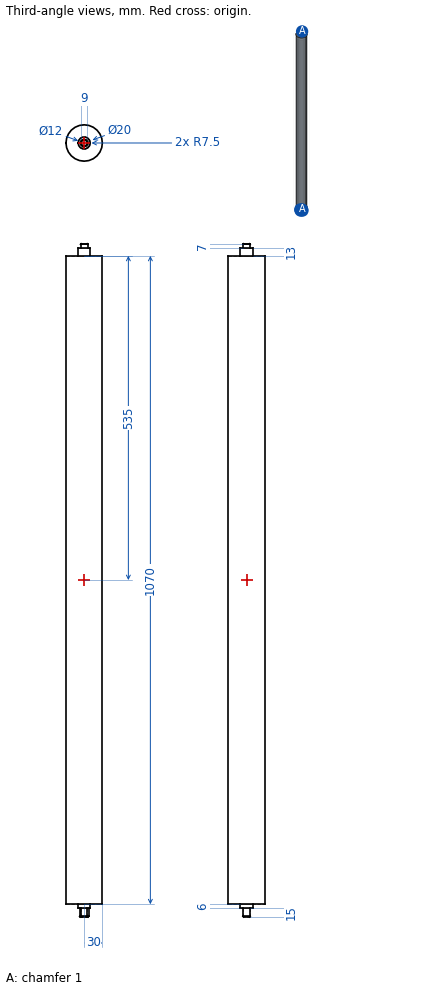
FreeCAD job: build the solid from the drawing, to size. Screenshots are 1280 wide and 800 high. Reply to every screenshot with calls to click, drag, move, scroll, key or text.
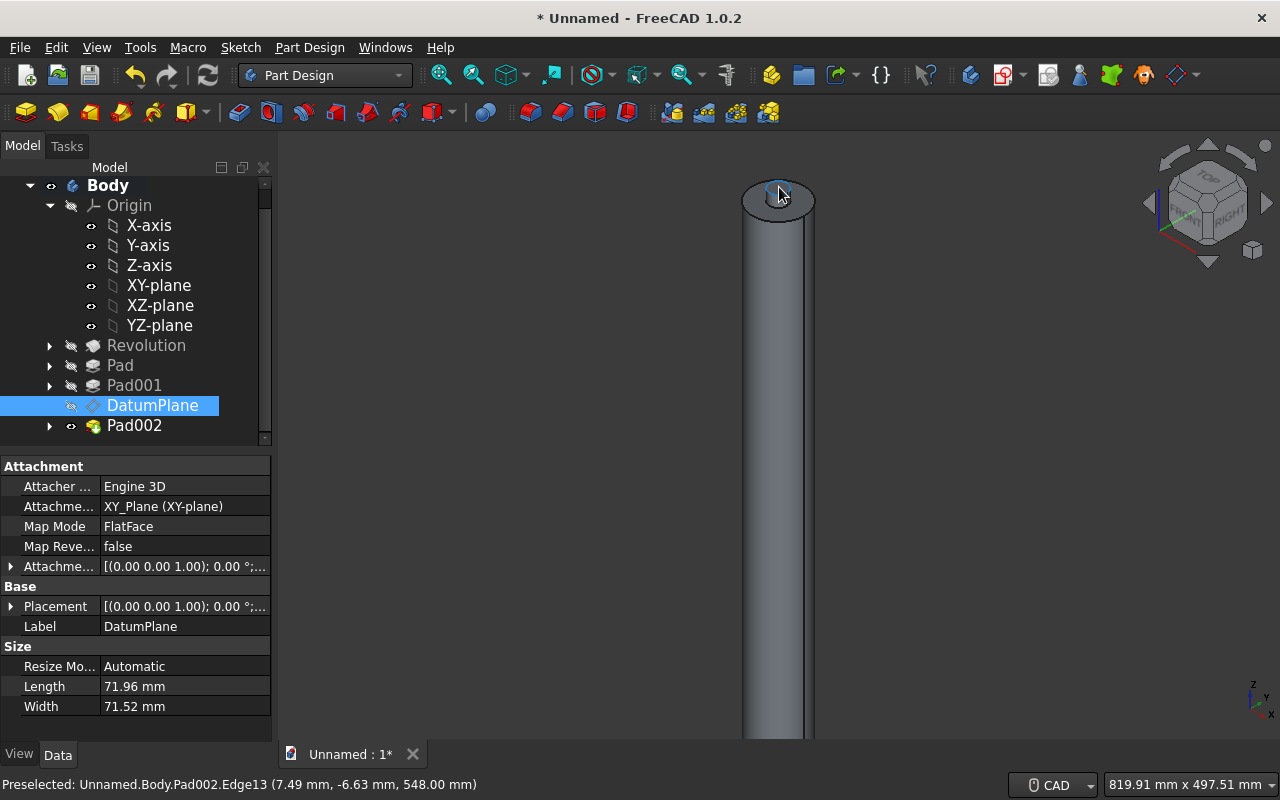
key(v)
key(f)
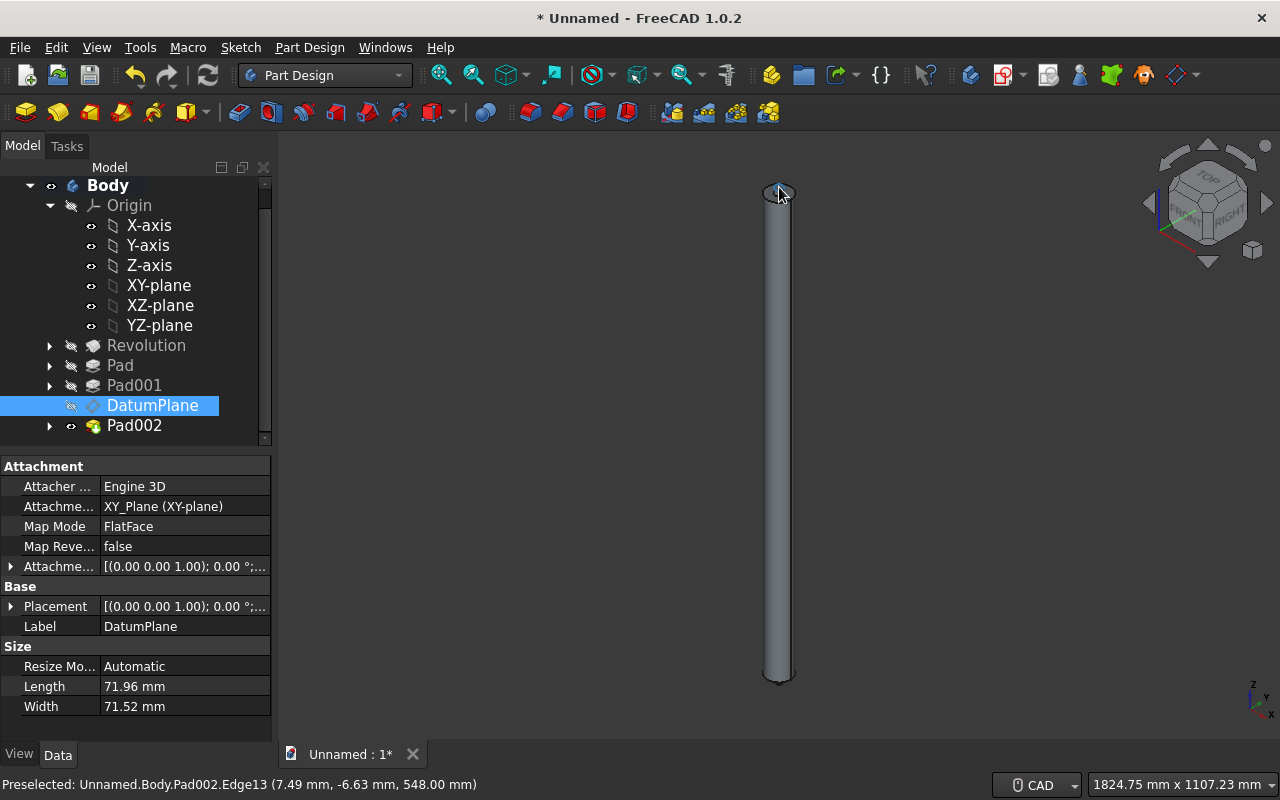
key(2)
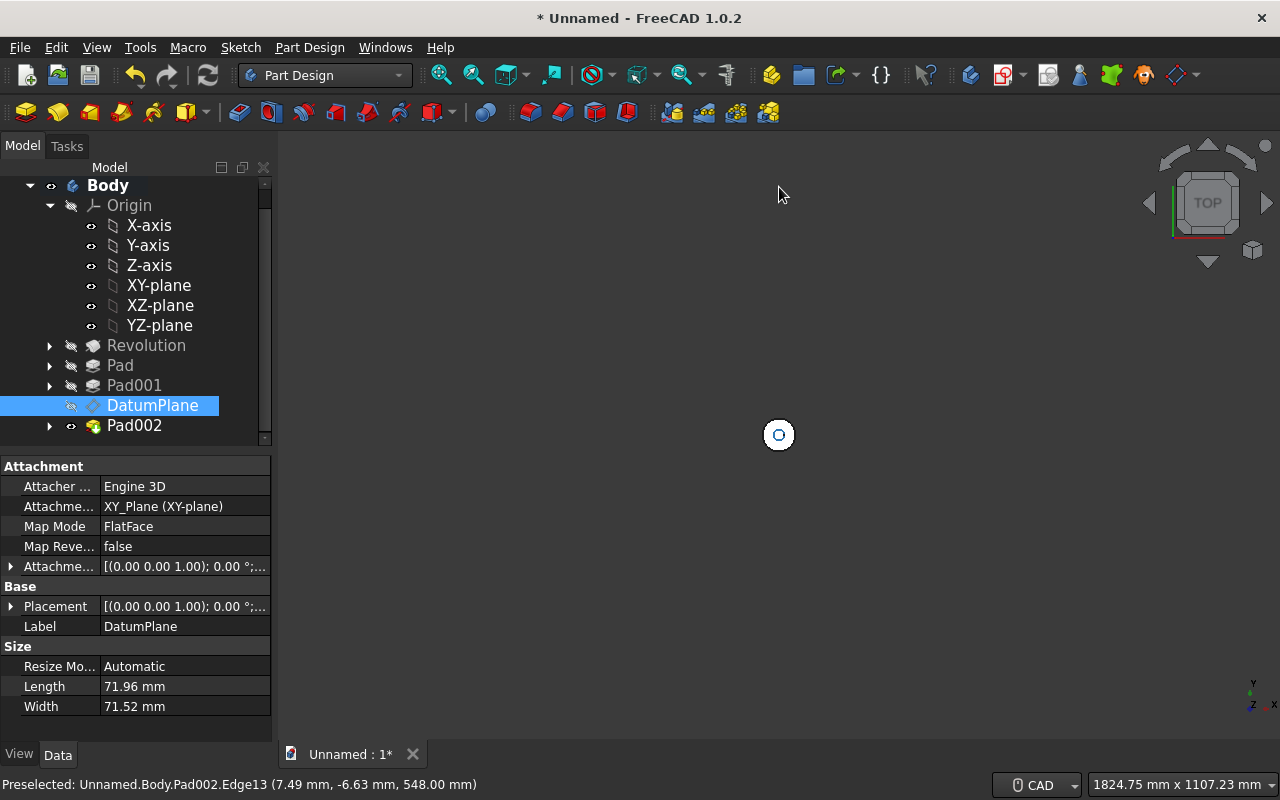
click(442, 76)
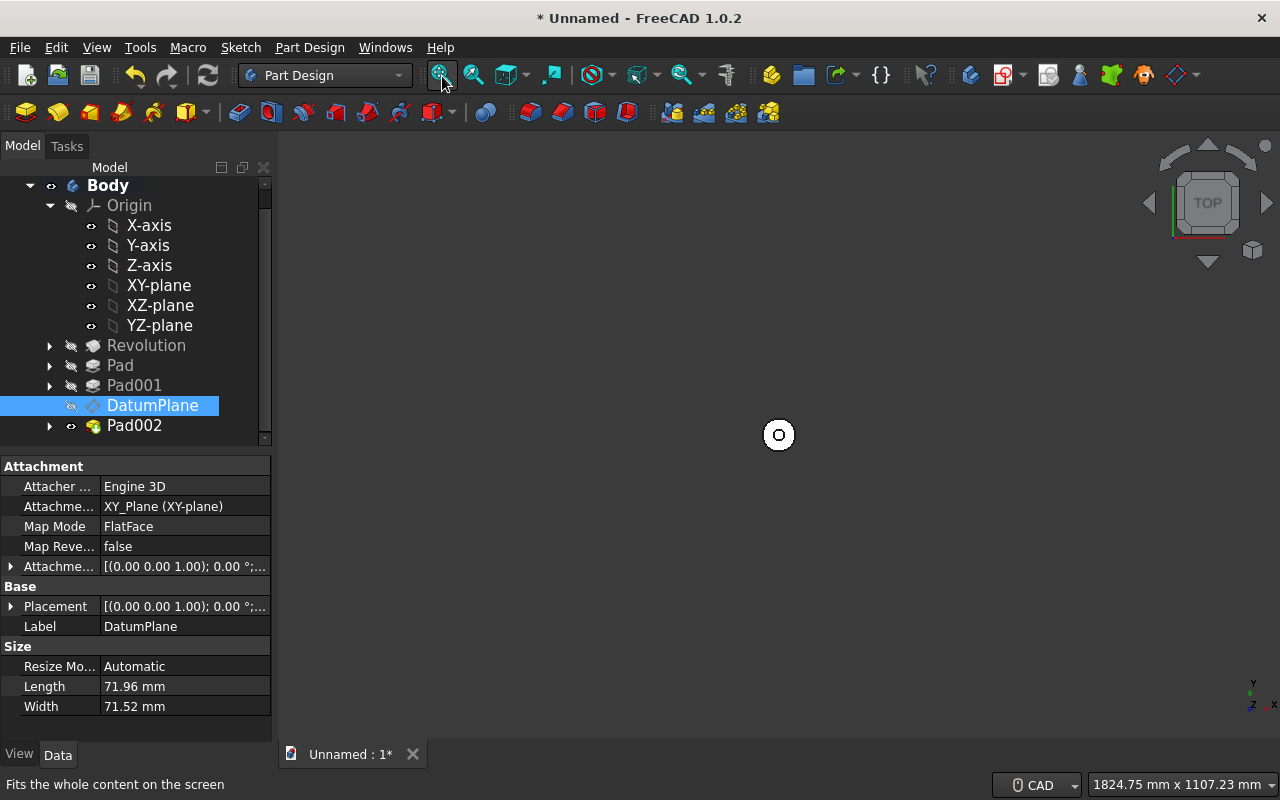
scroll(779, 434, up, 4)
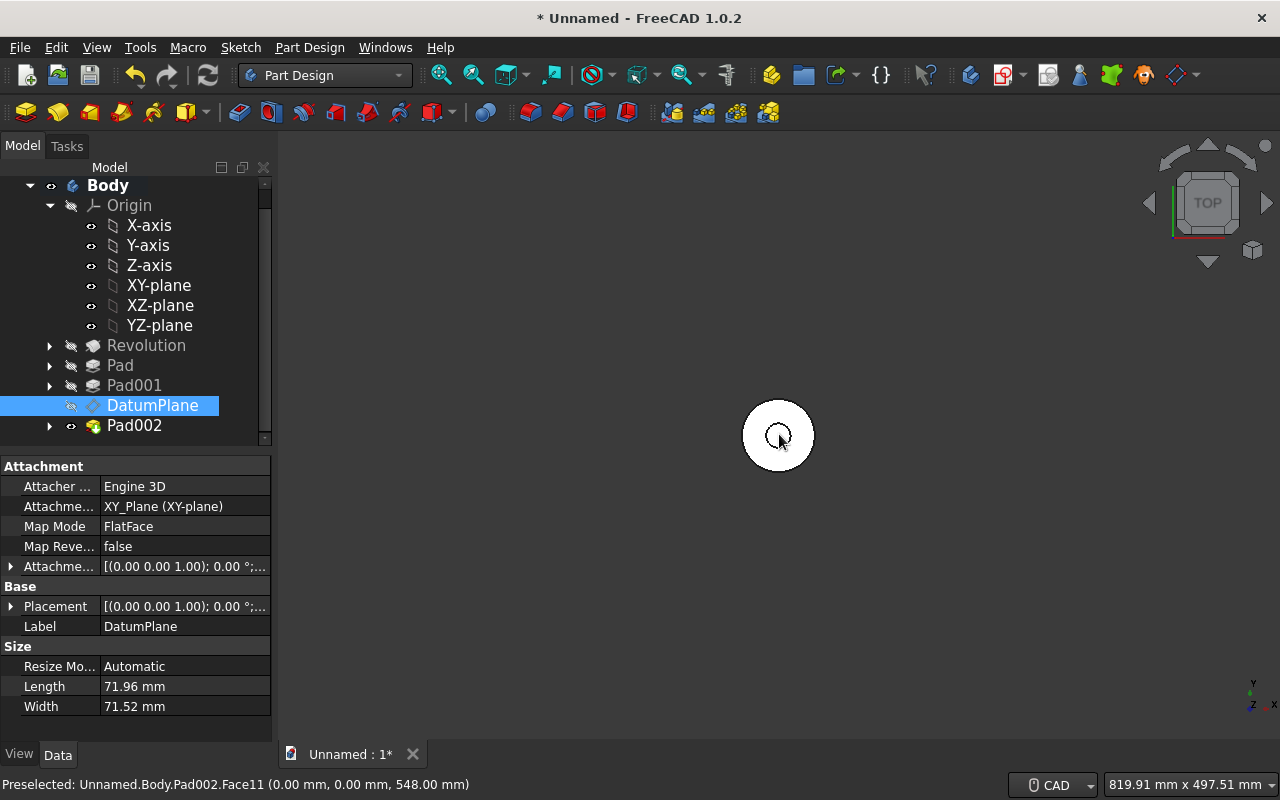
click(778, 435)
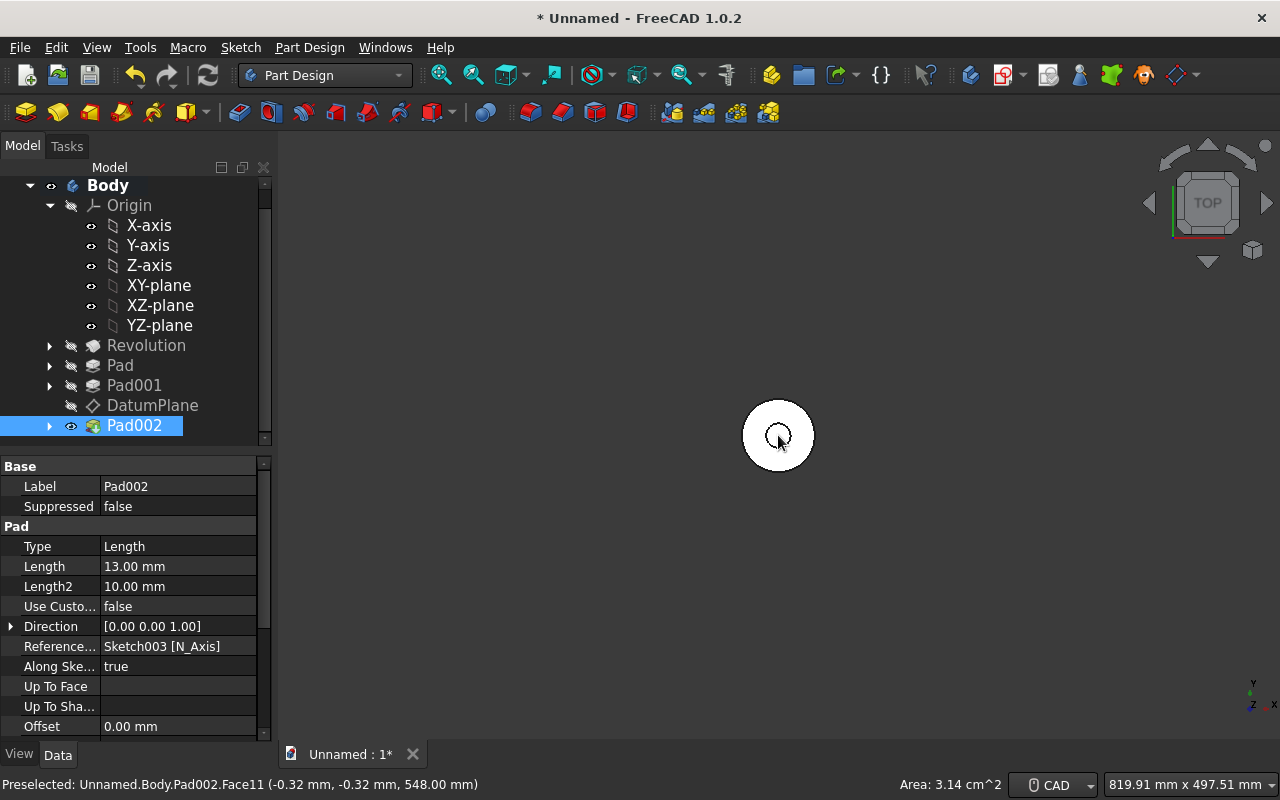
click(1004, 76)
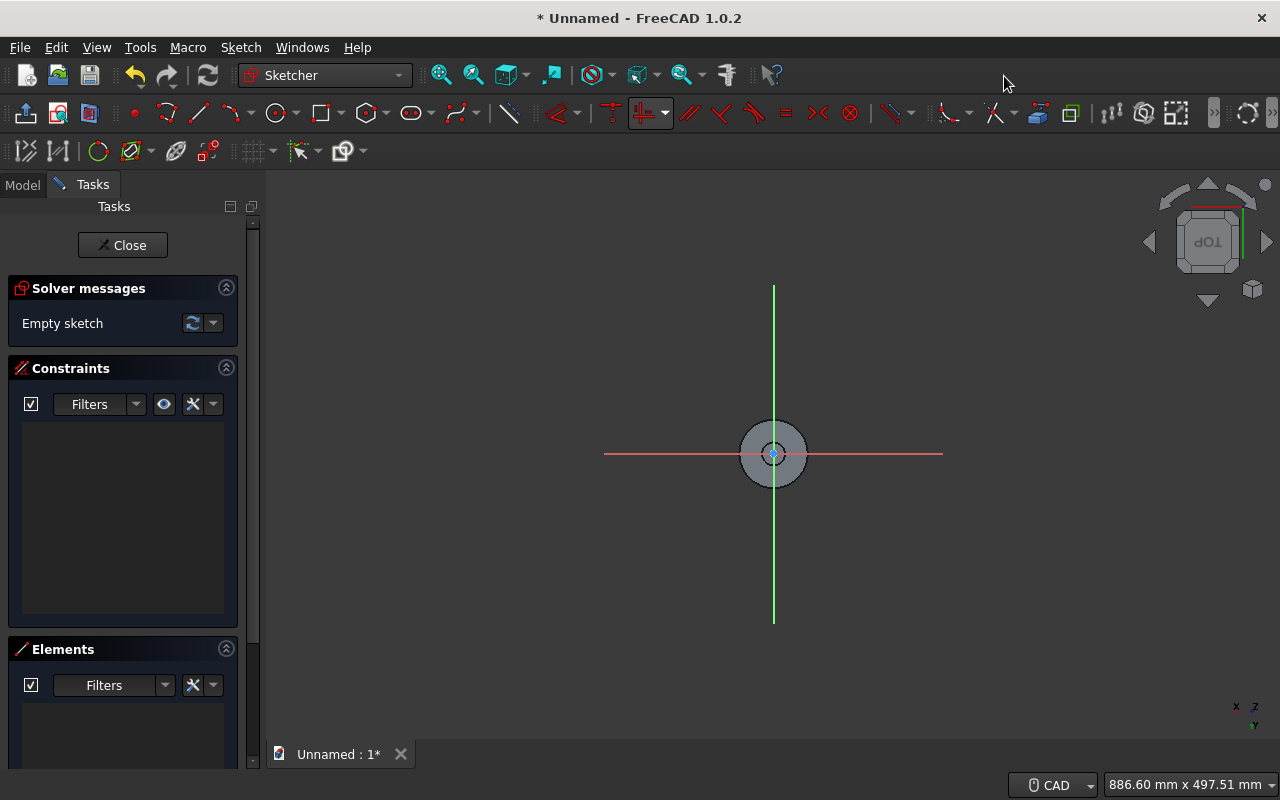
scroll(777, 454, up, 15)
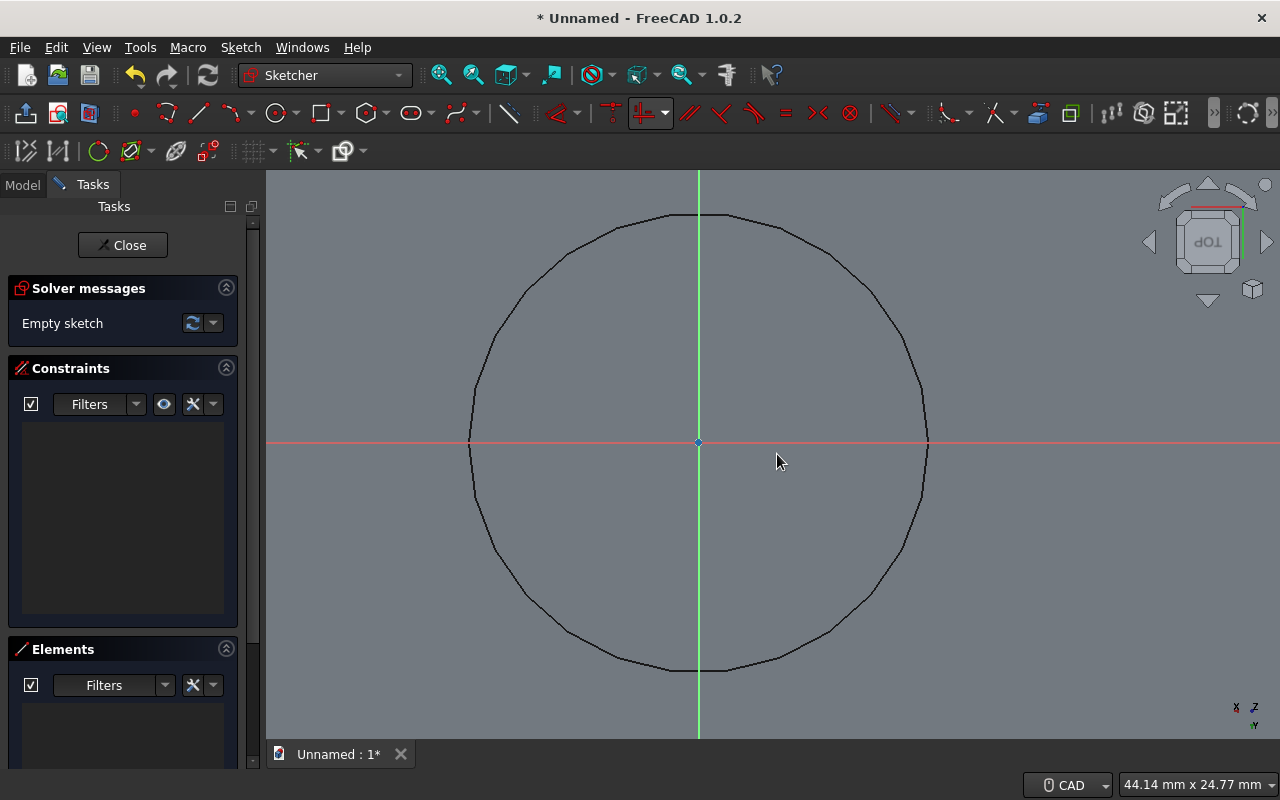
key(g)
key(c)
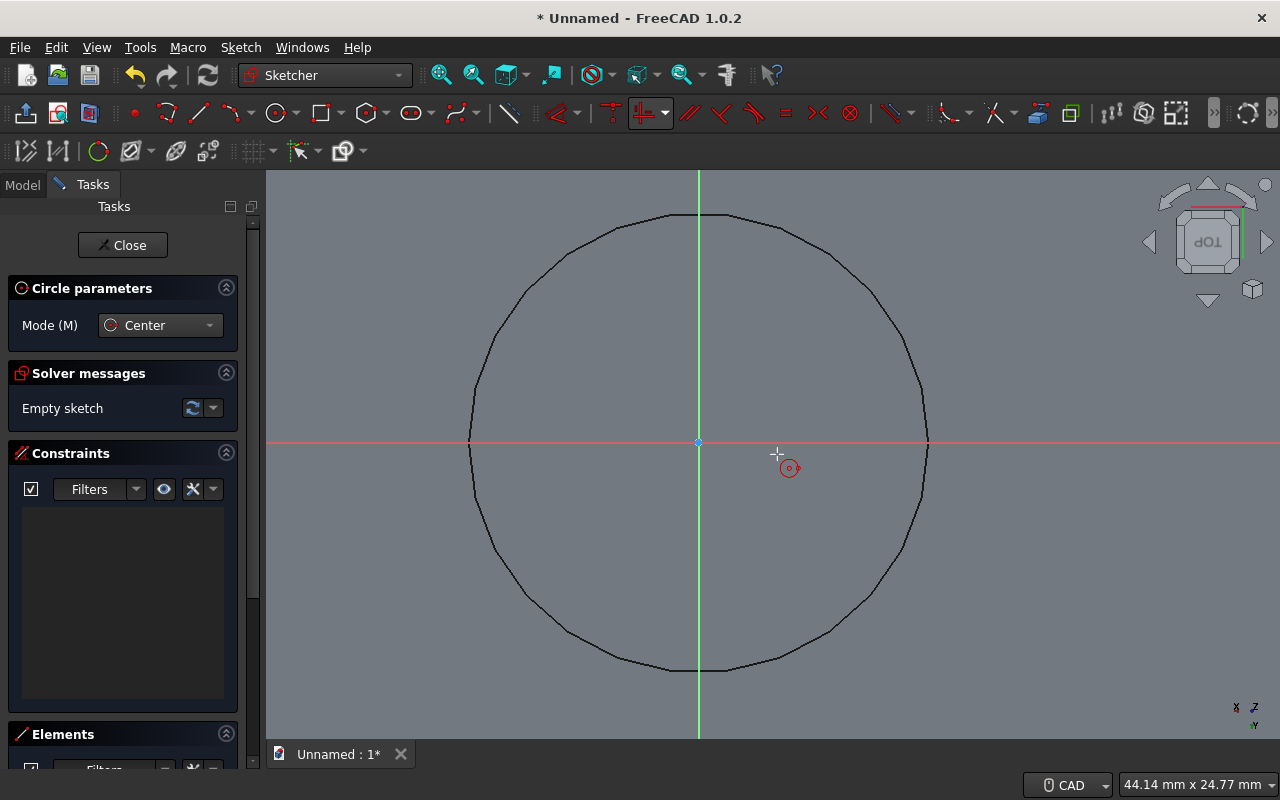
click(699, 443)
move(796, 346)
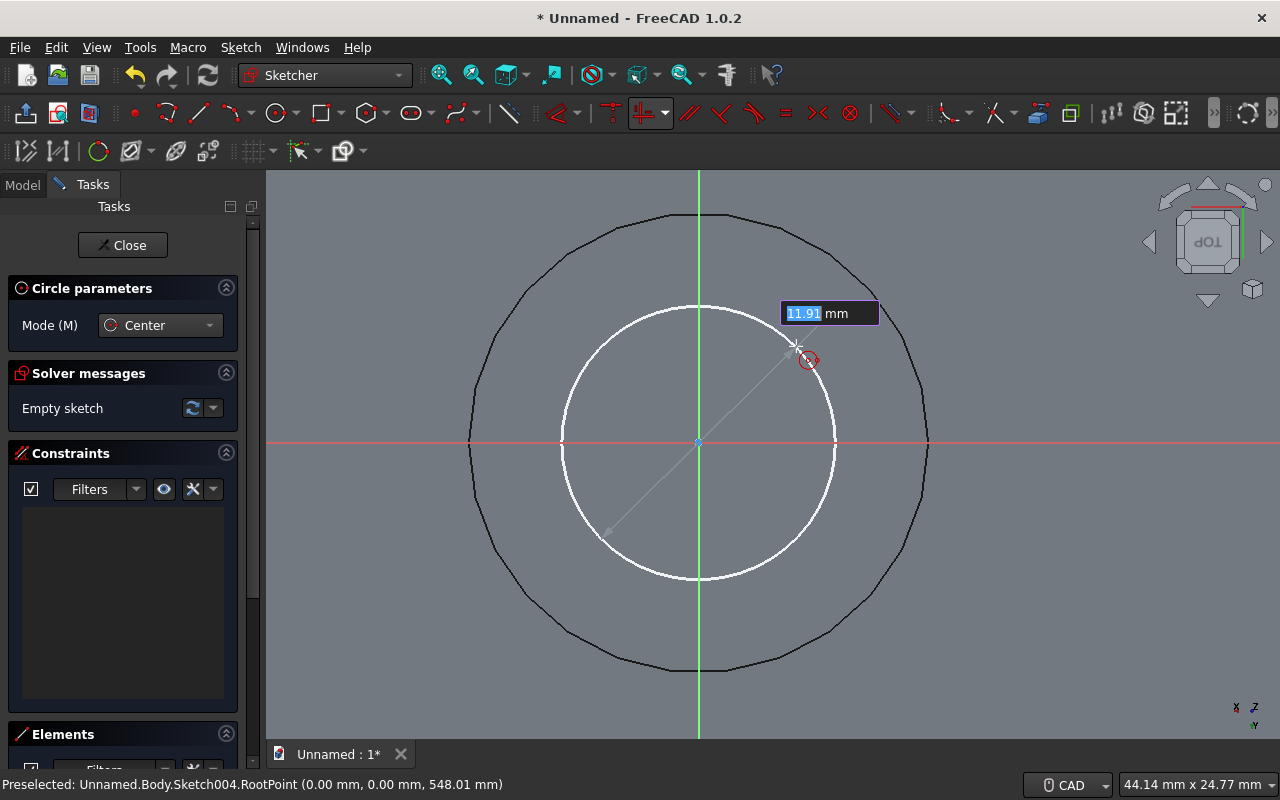
text(12)
key(Return)
key(Escape)